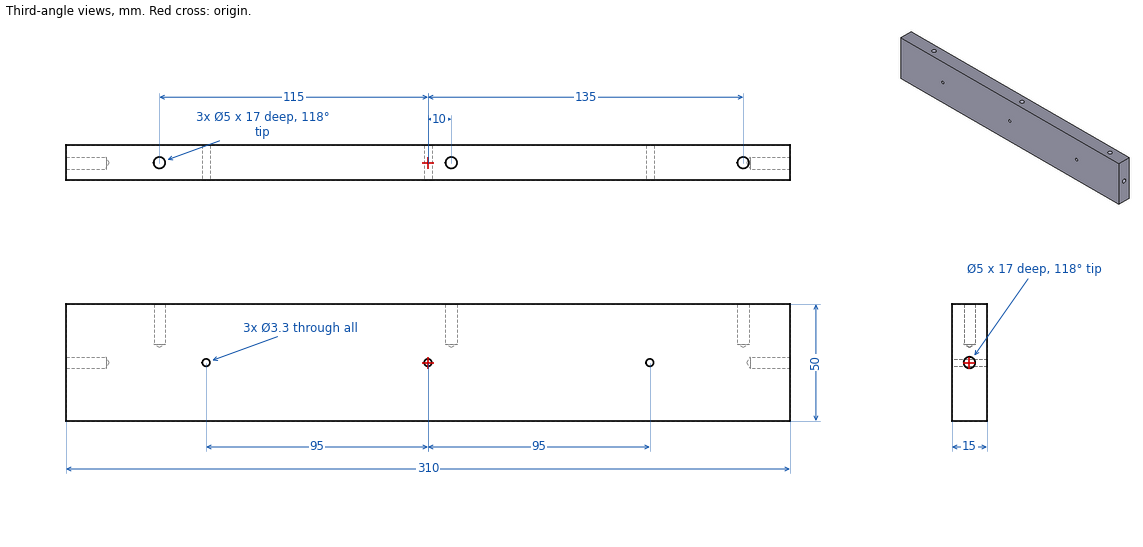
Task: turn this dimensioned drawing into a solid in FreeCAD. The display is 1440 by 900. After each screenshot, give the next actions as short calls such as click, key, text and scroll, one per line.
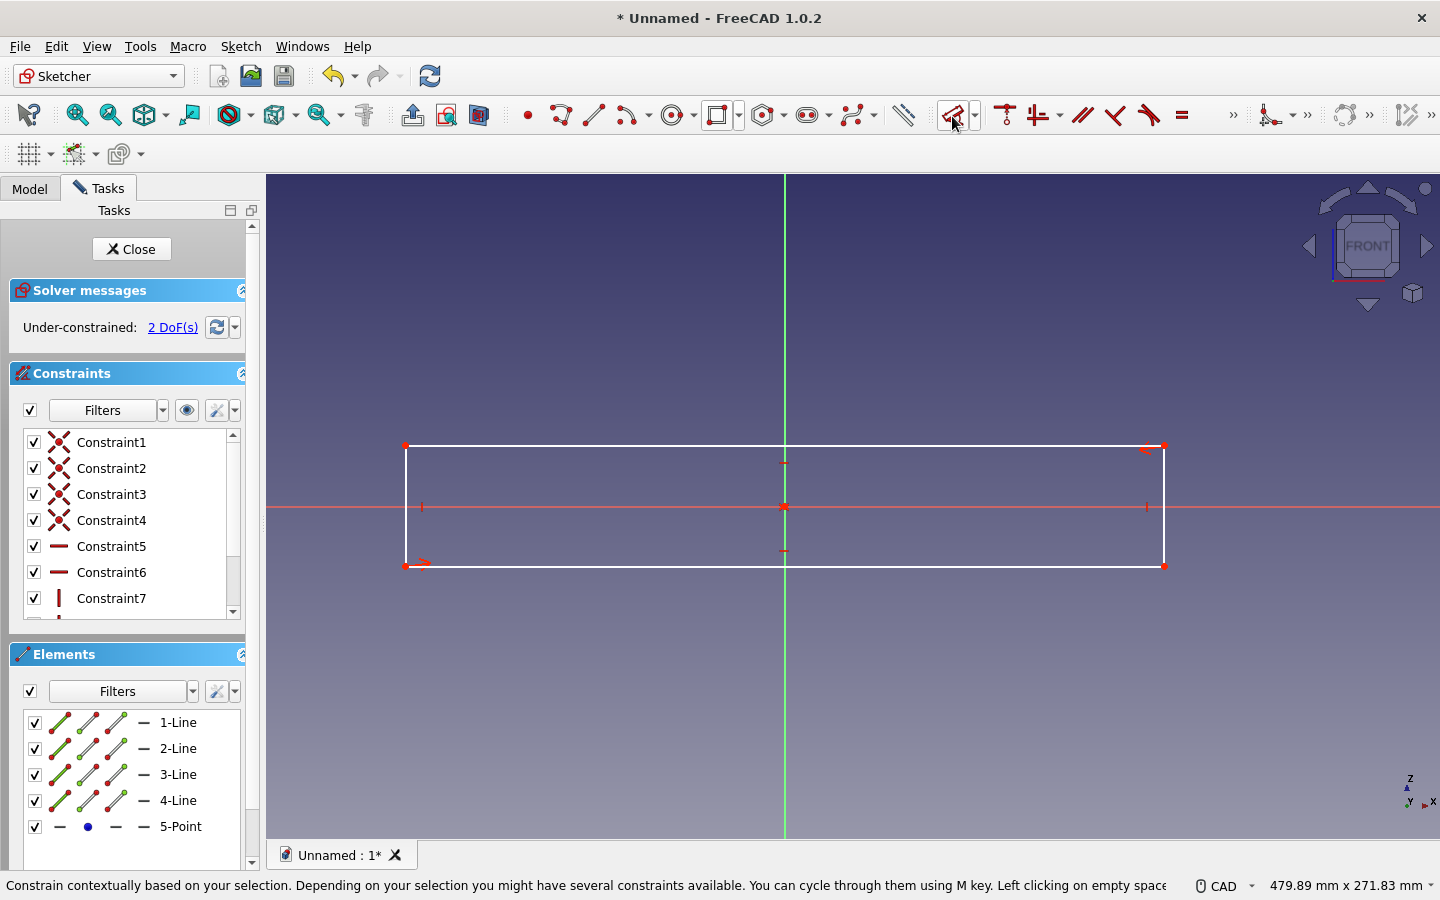
click(1164, 531)
click(1198, 479)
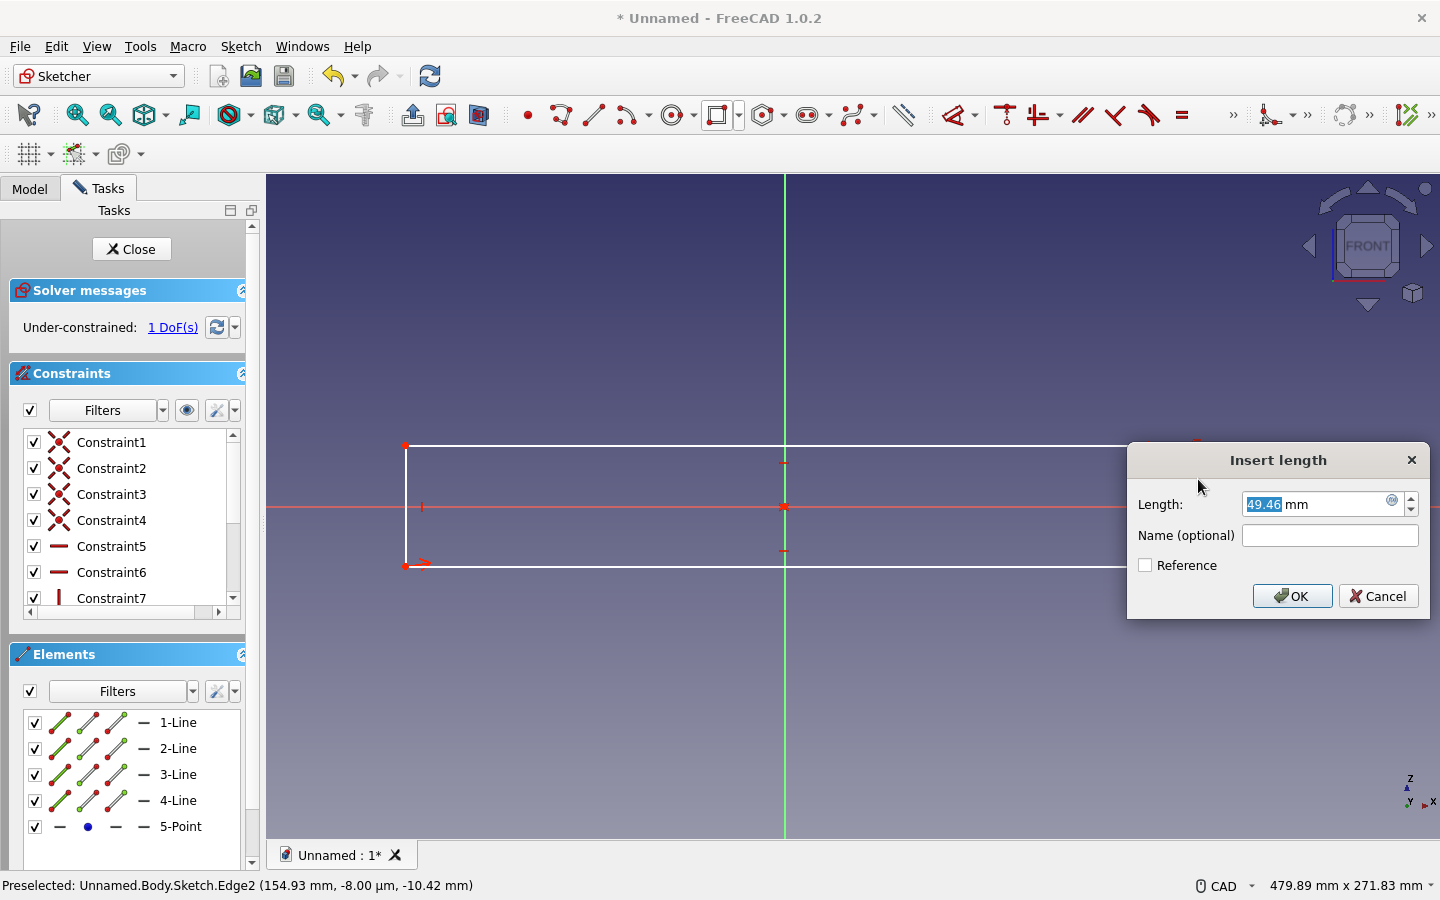
text(50)
key(Return)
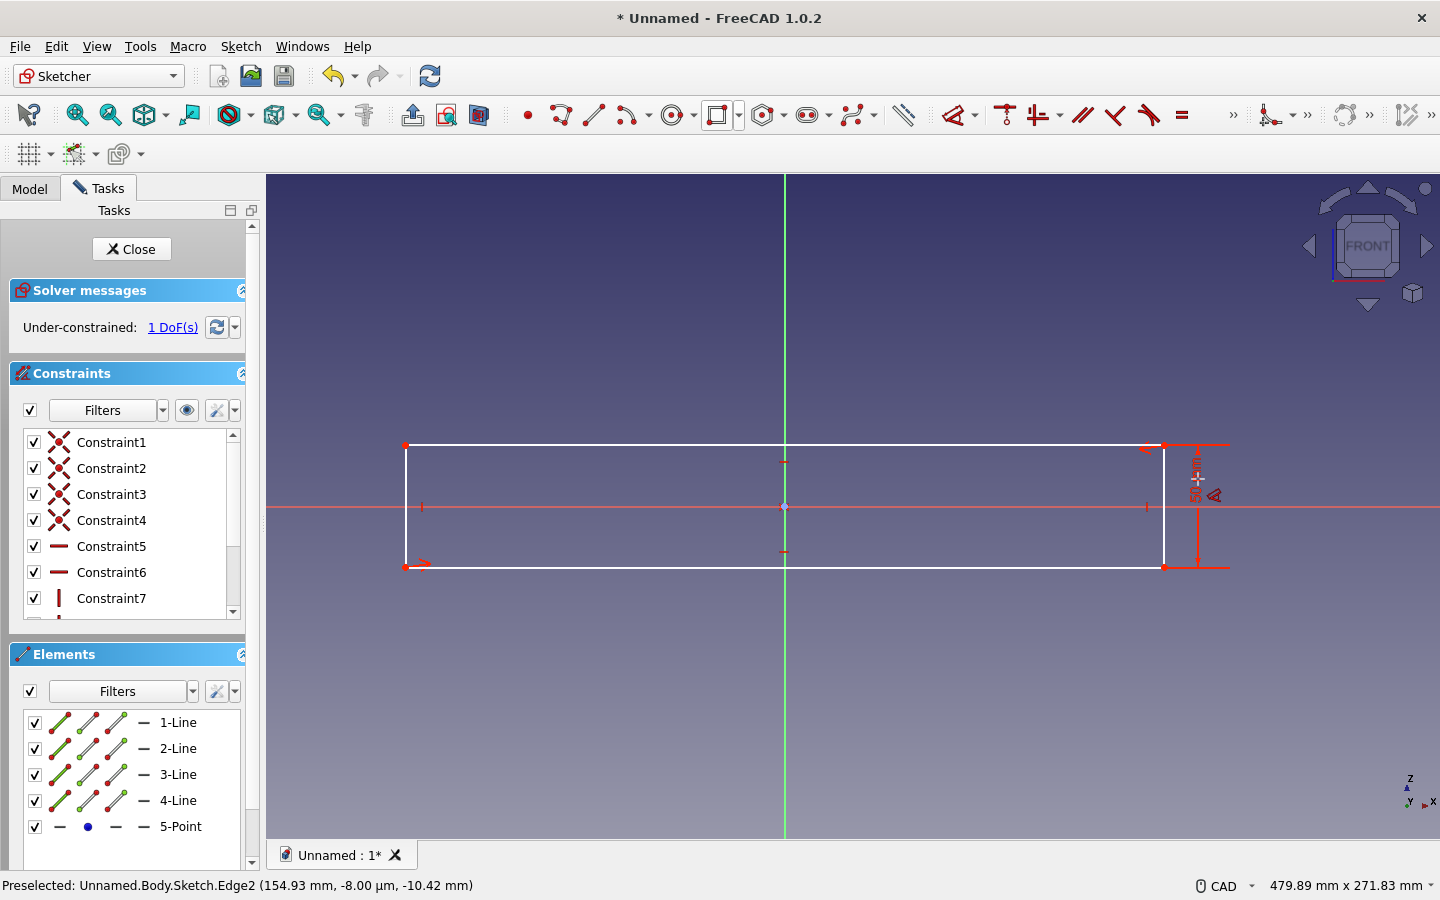
click(633, 568)
click(611, 602)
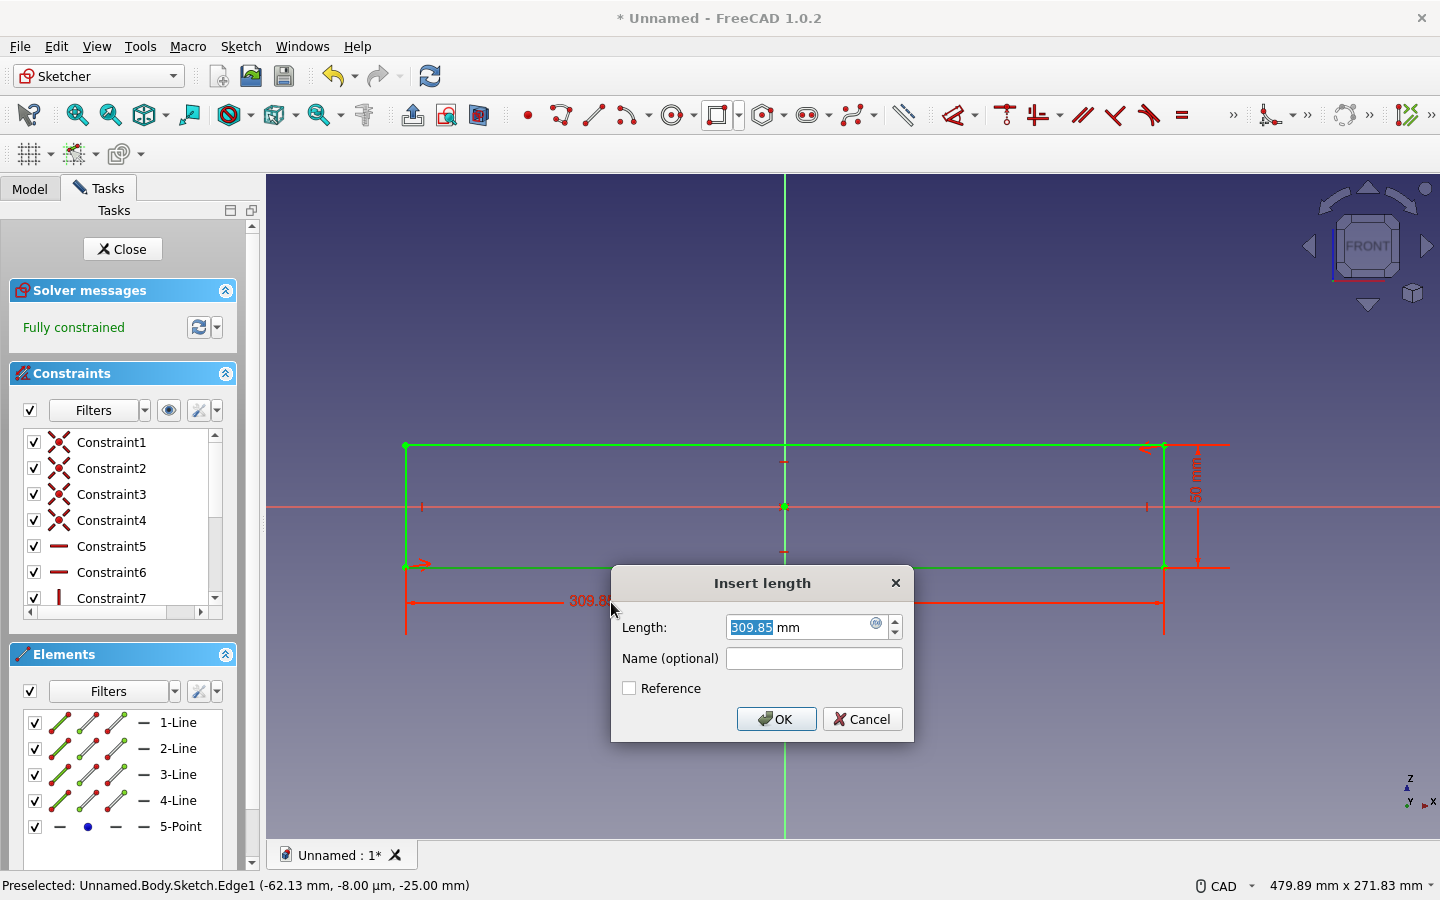
text(310)
key(Return)
key(Escape)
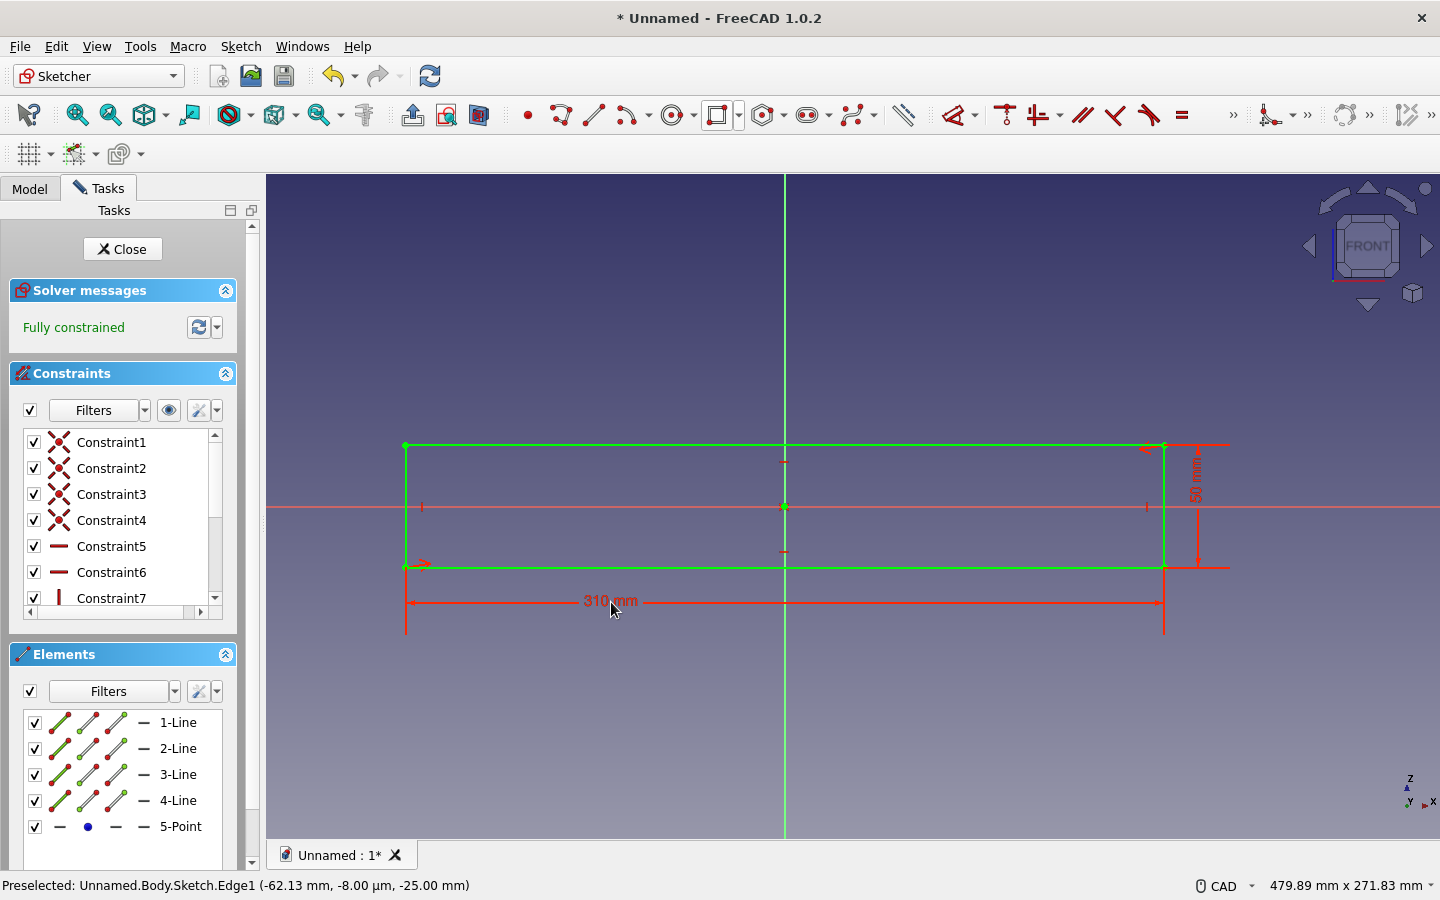
click(123, 249)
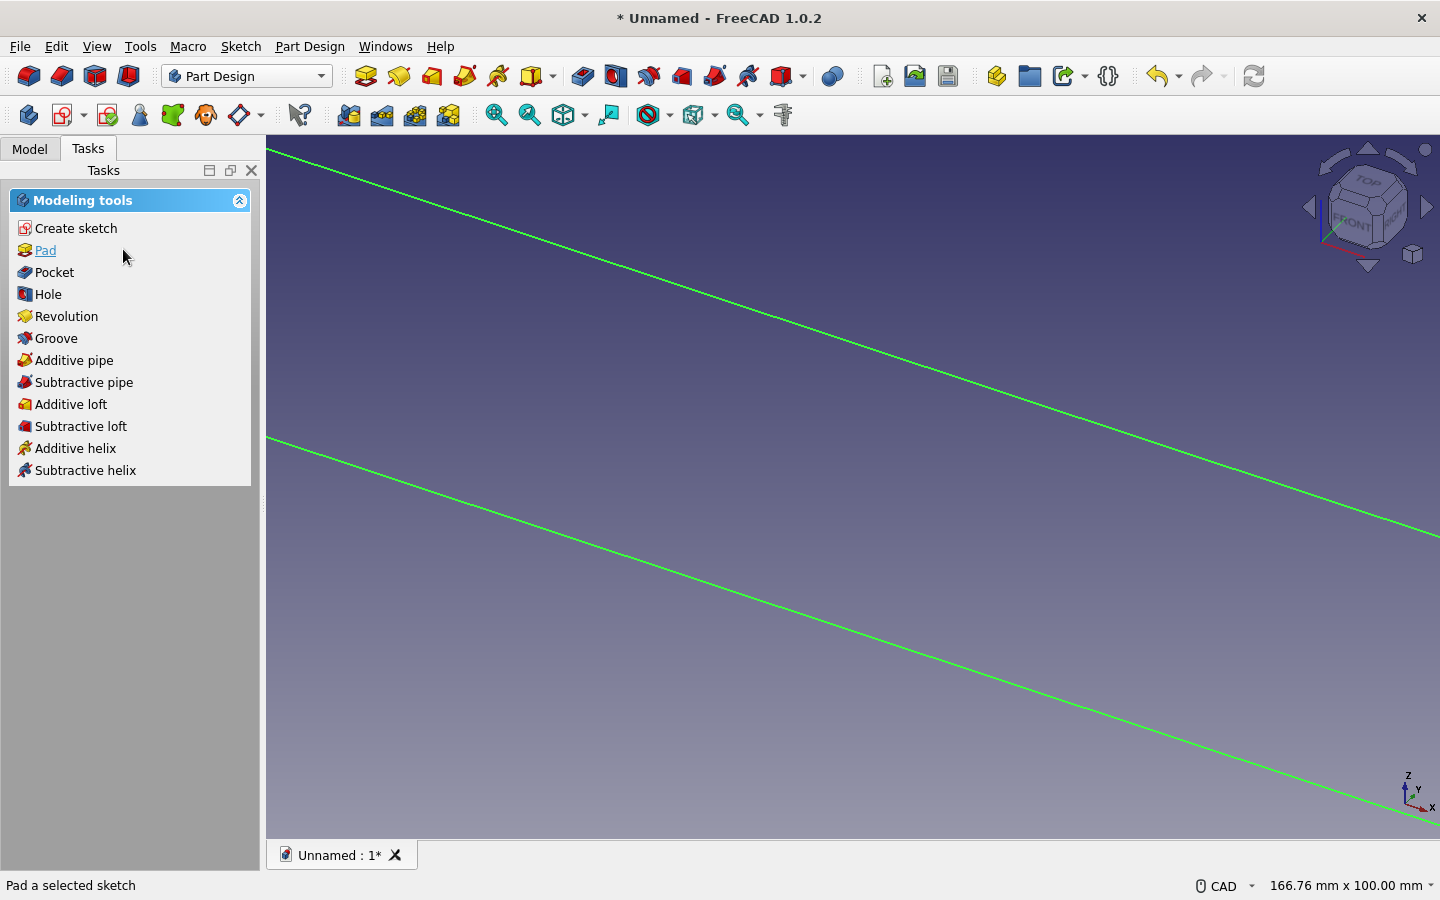
click(366, 76)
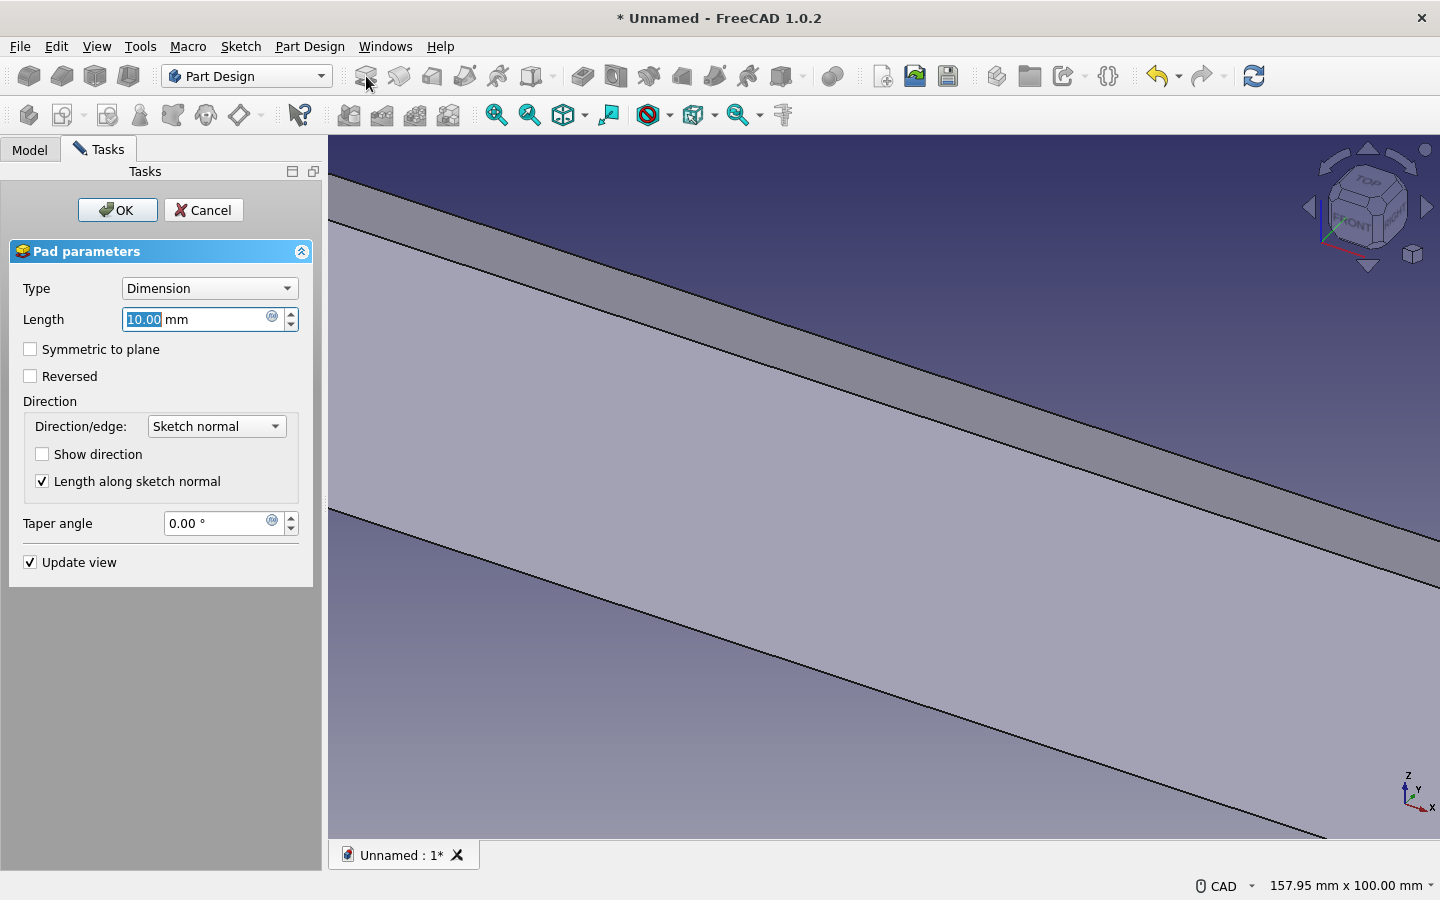
text(15)
key(Tab)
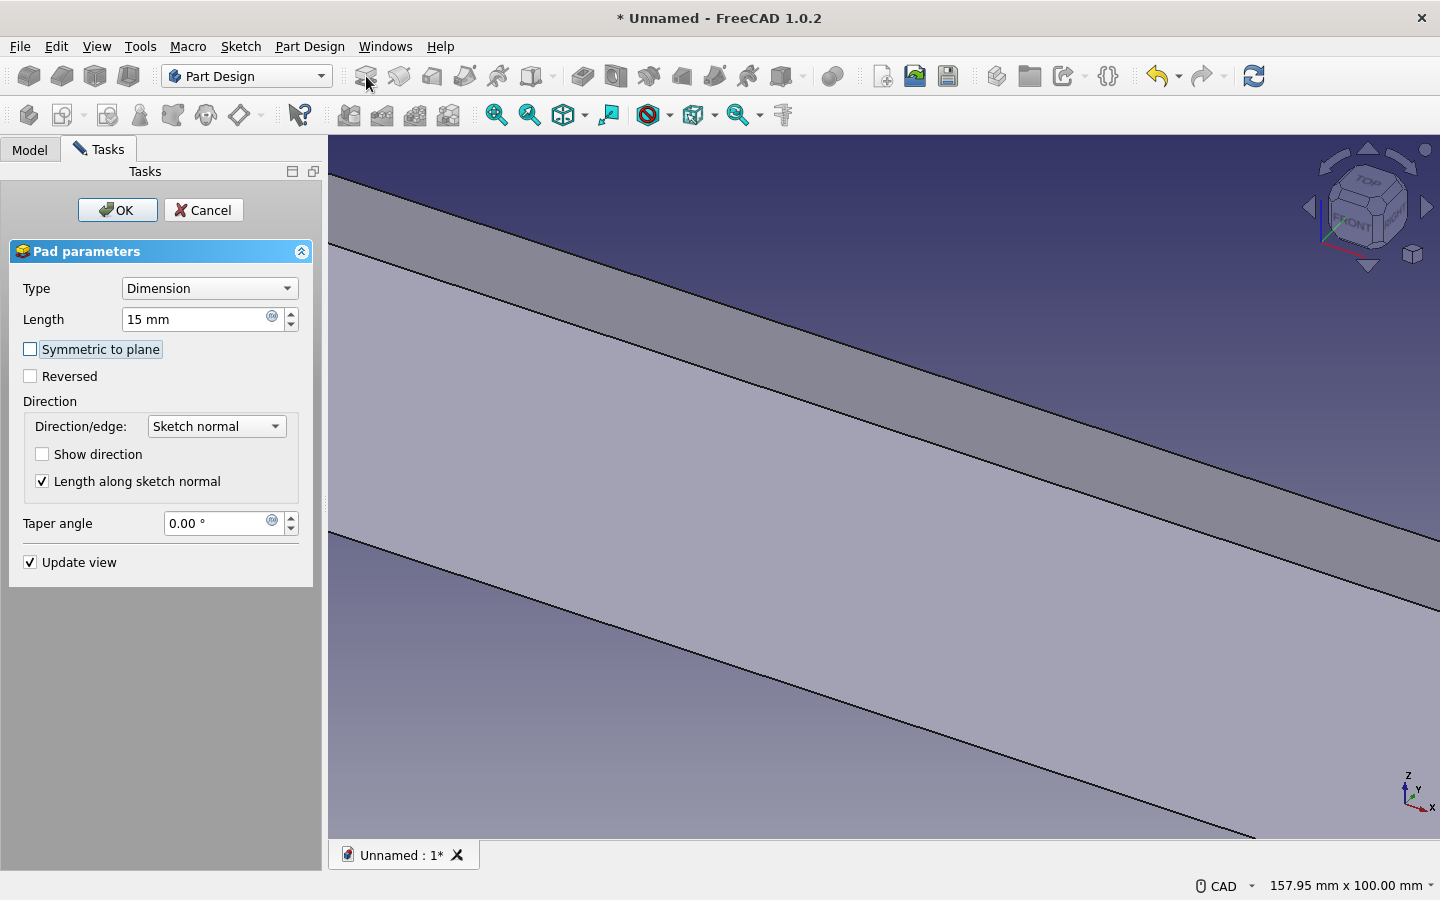
click(31, 349)